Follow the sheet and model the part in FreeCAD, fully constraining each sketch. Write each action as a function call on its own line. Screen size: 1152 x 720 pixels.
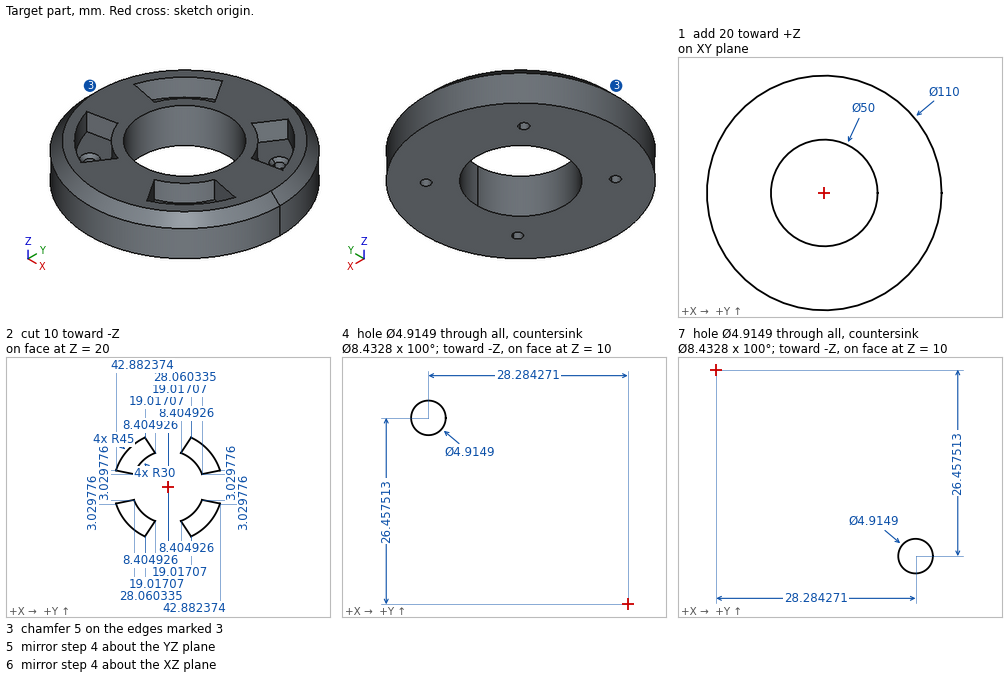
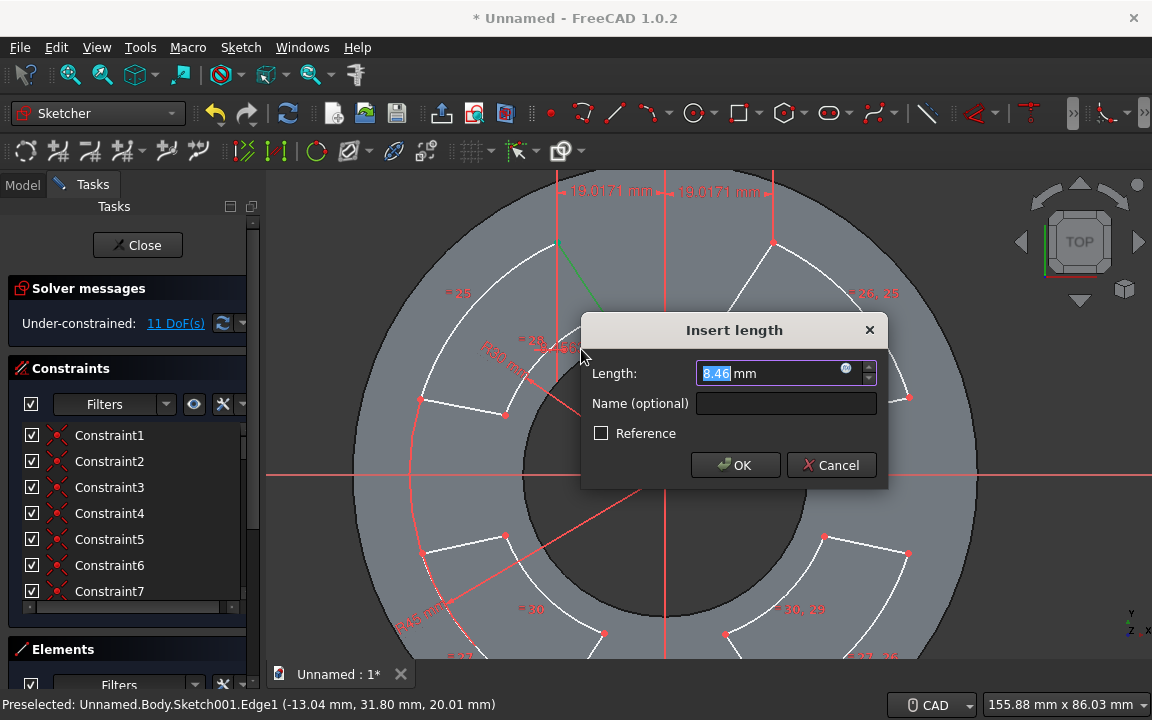
text(8.404926)
key(Return)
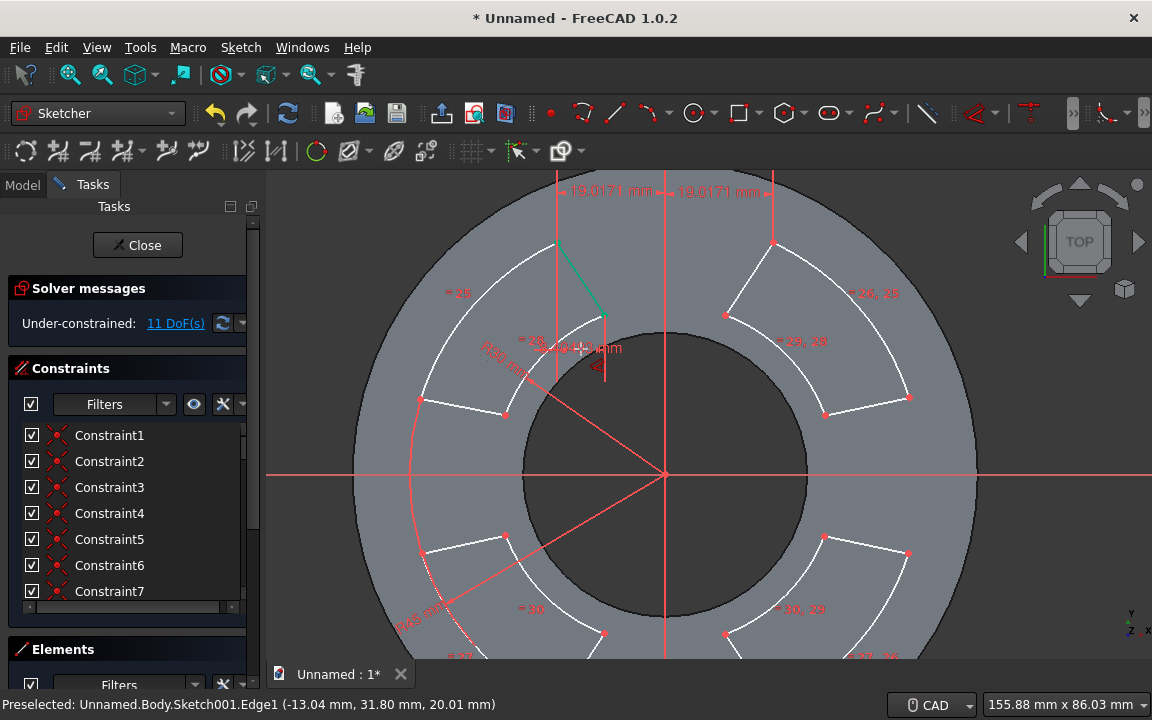
scroll(446, 404, up, 5)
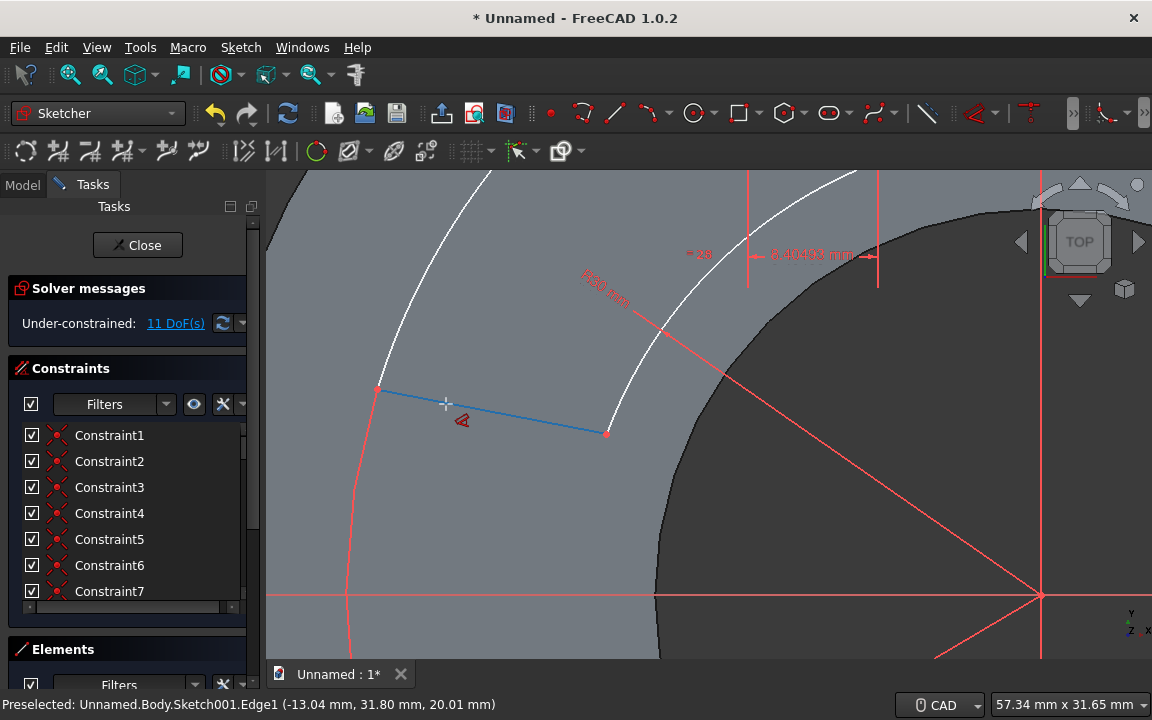
click(446, 403)
click(343, 412)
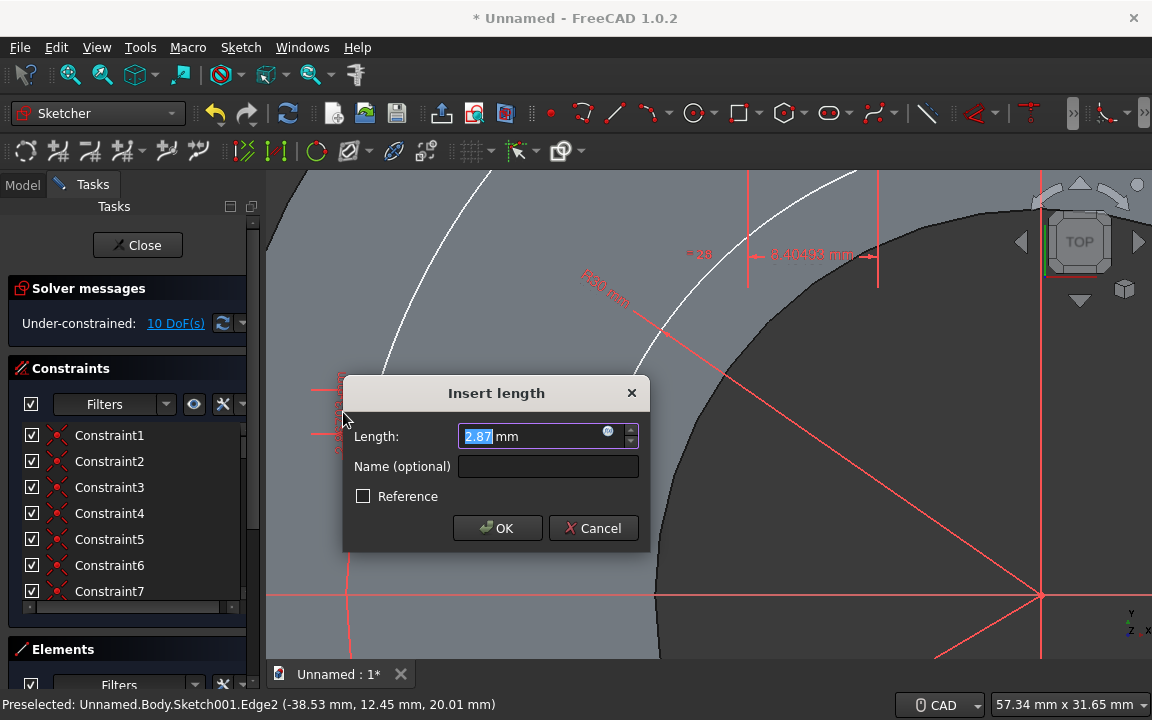
text(3.029776)
key(Return)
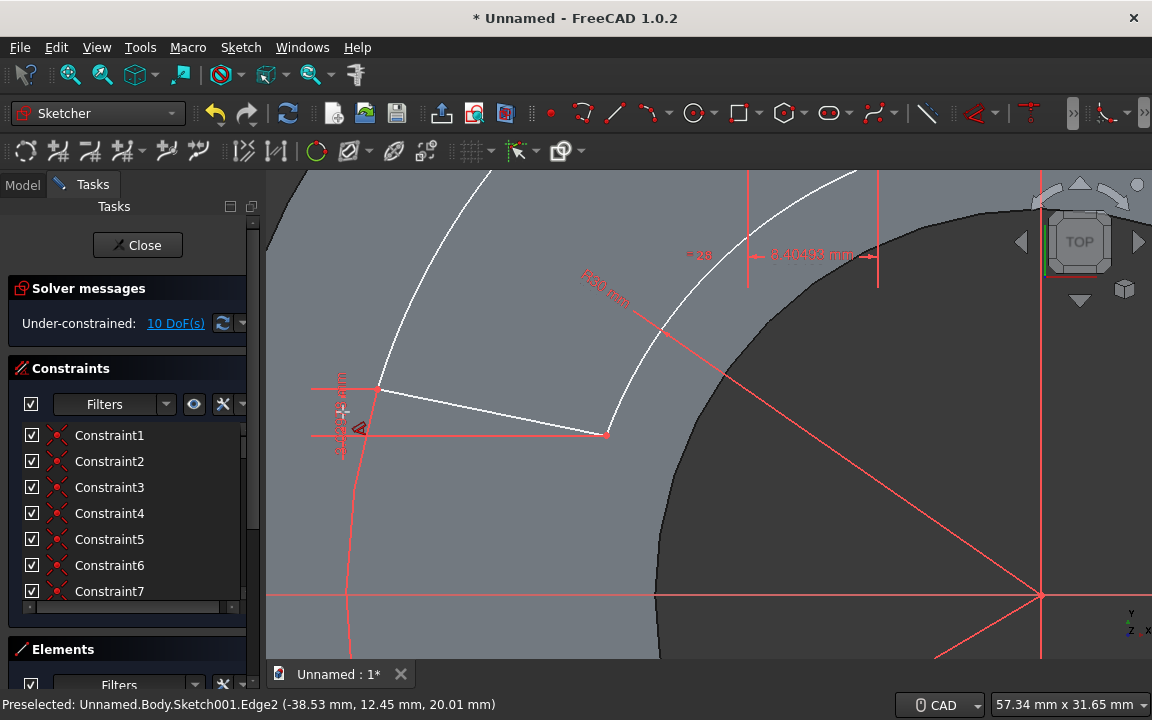
scroll(509, 355, down, 7)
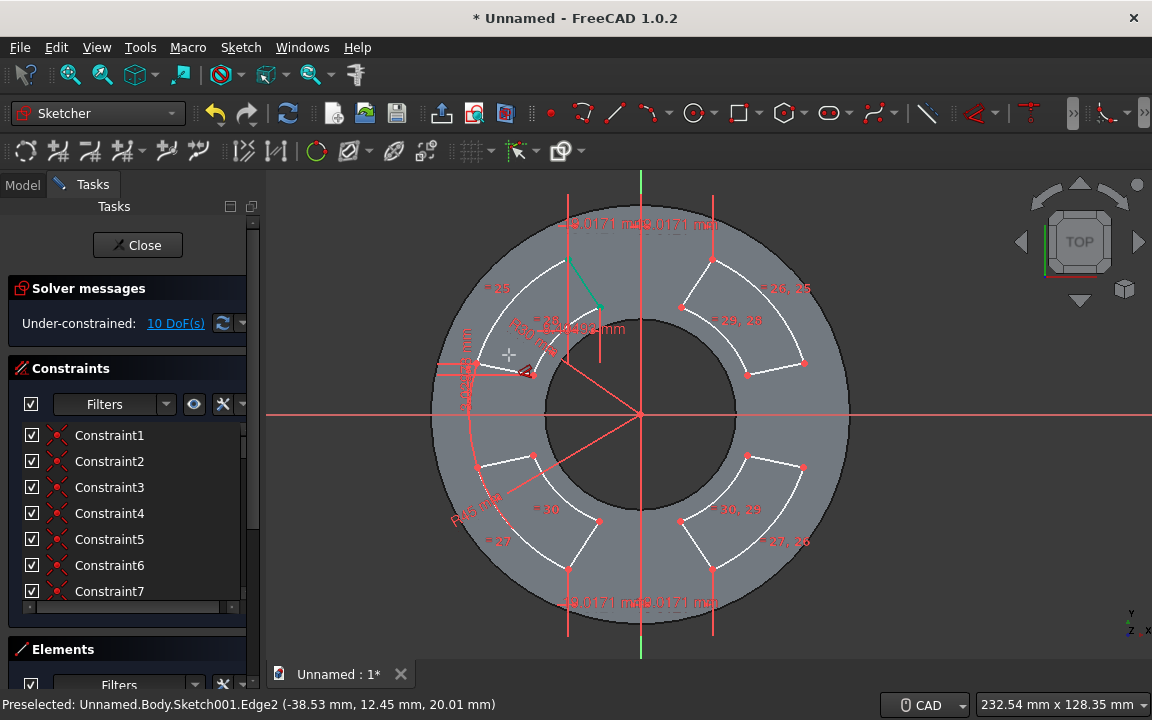
scroll(765, 371, up, 7)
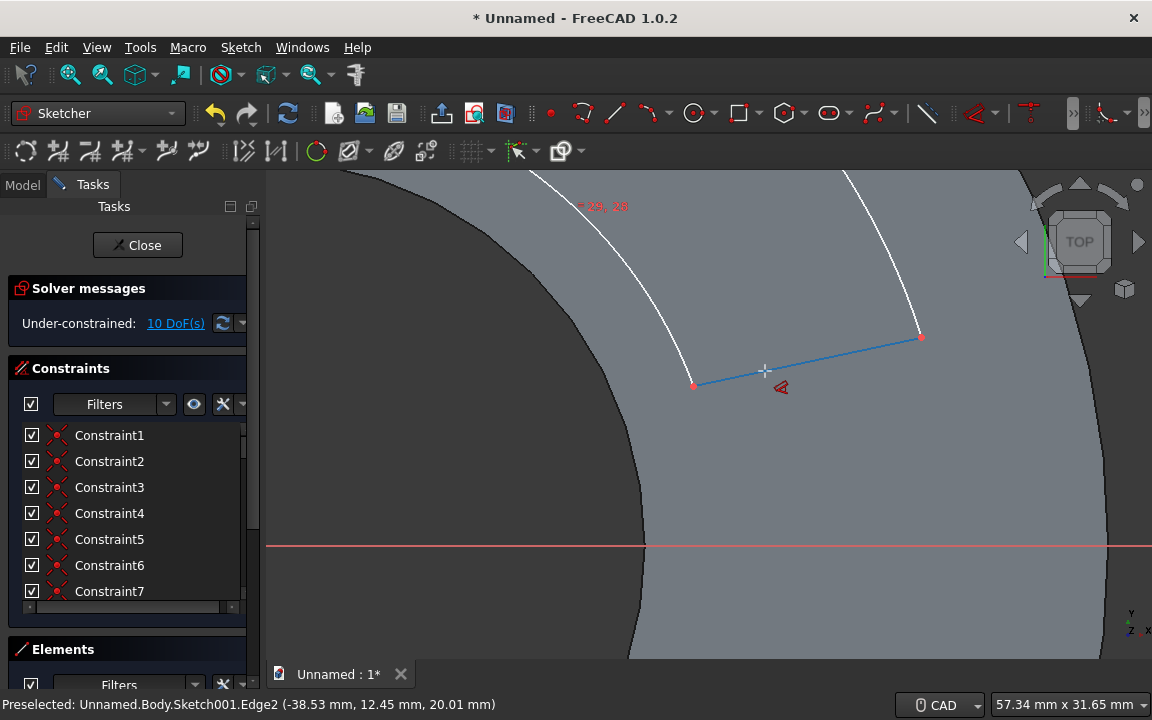
click(762, 372)
click(956, 362)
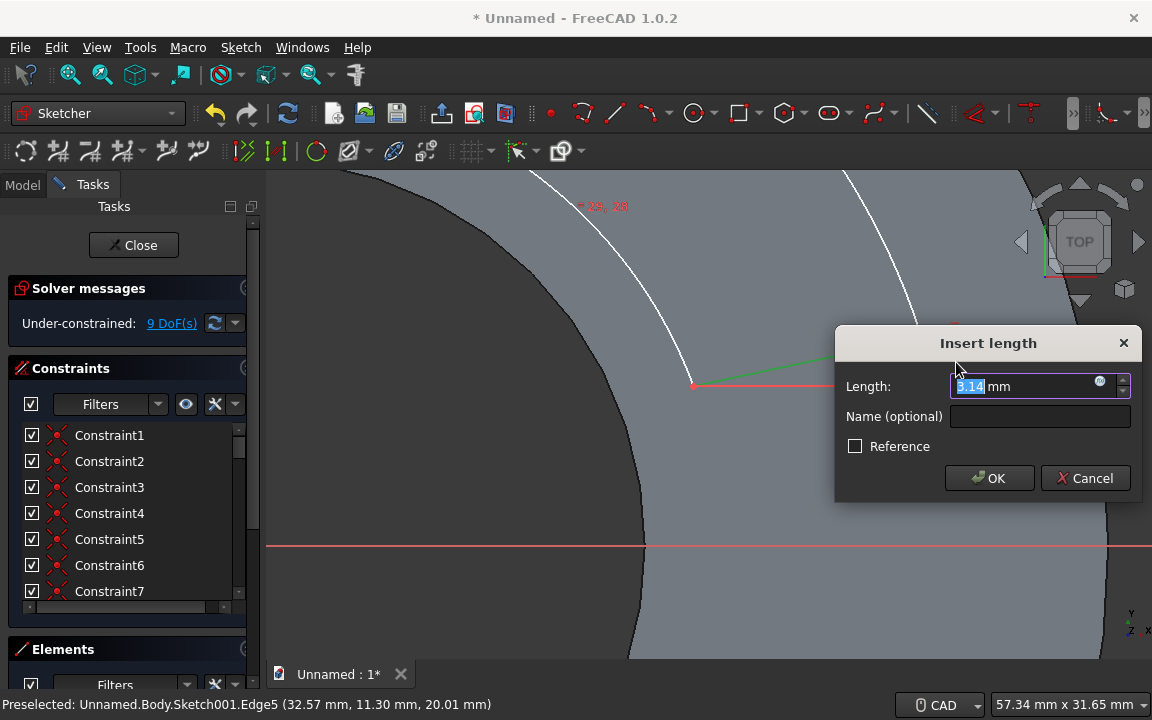
text(3.029776)
key(Return)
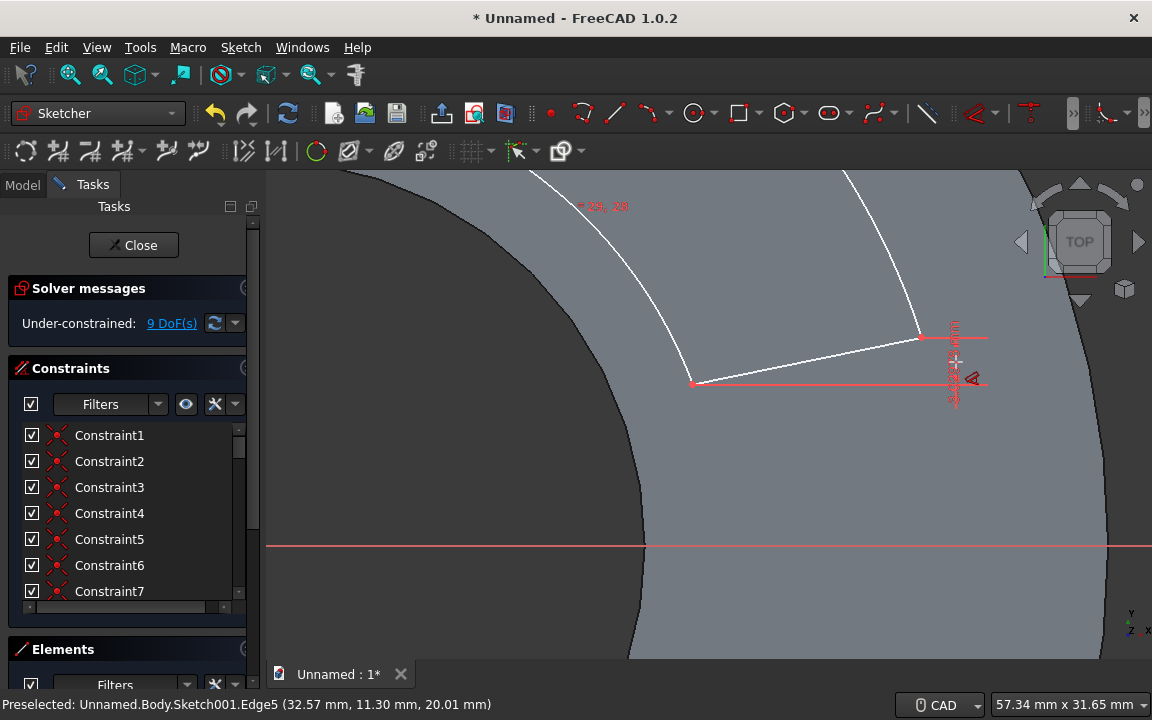
scroll(766, 371, down, 7)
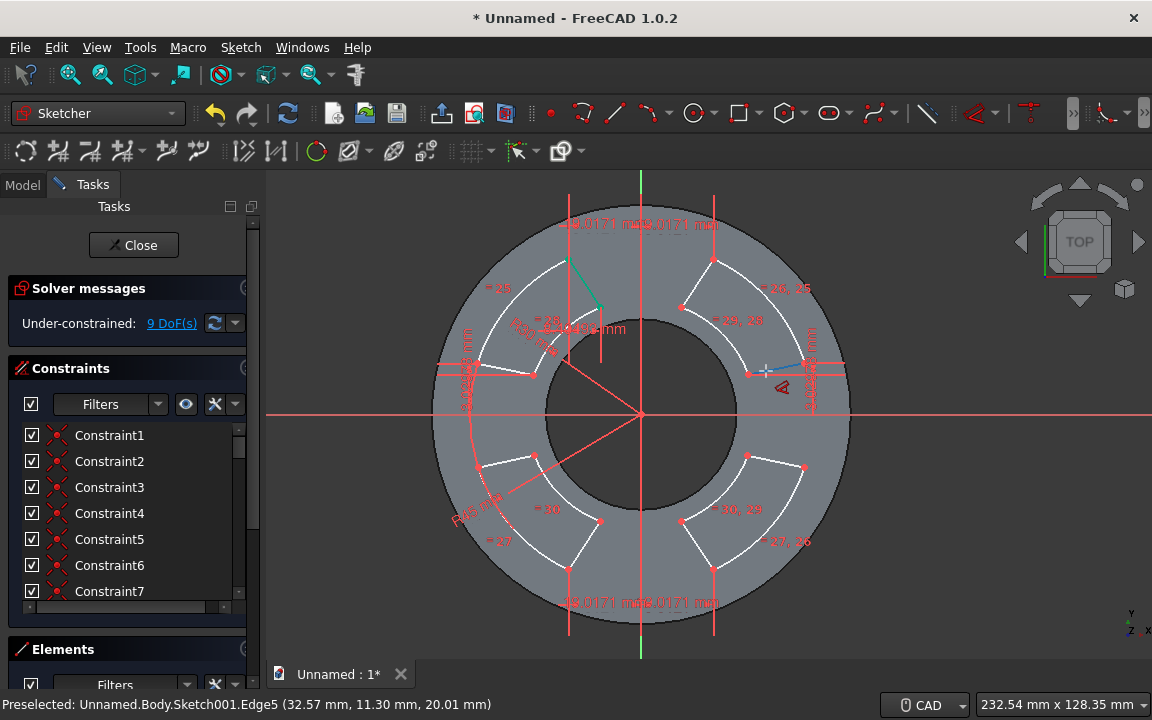
scroll(704, 274, up, 2)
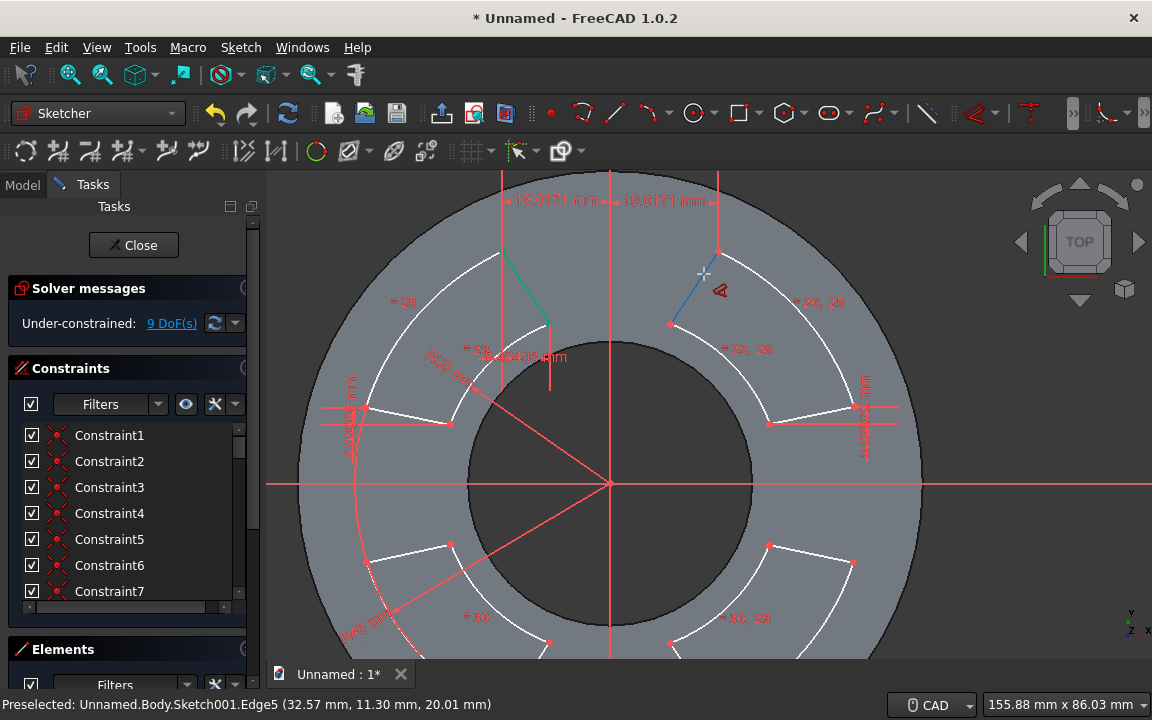
click(704, 273)
click(695, 358)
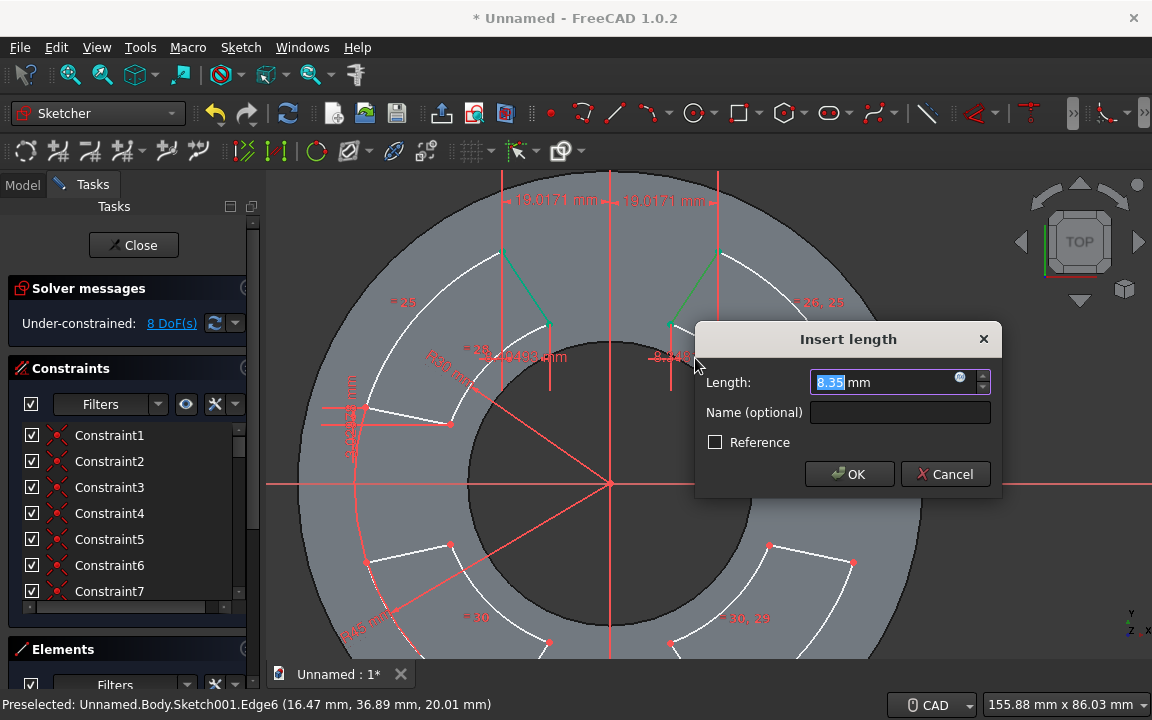
text(8.404926)
key(Return)